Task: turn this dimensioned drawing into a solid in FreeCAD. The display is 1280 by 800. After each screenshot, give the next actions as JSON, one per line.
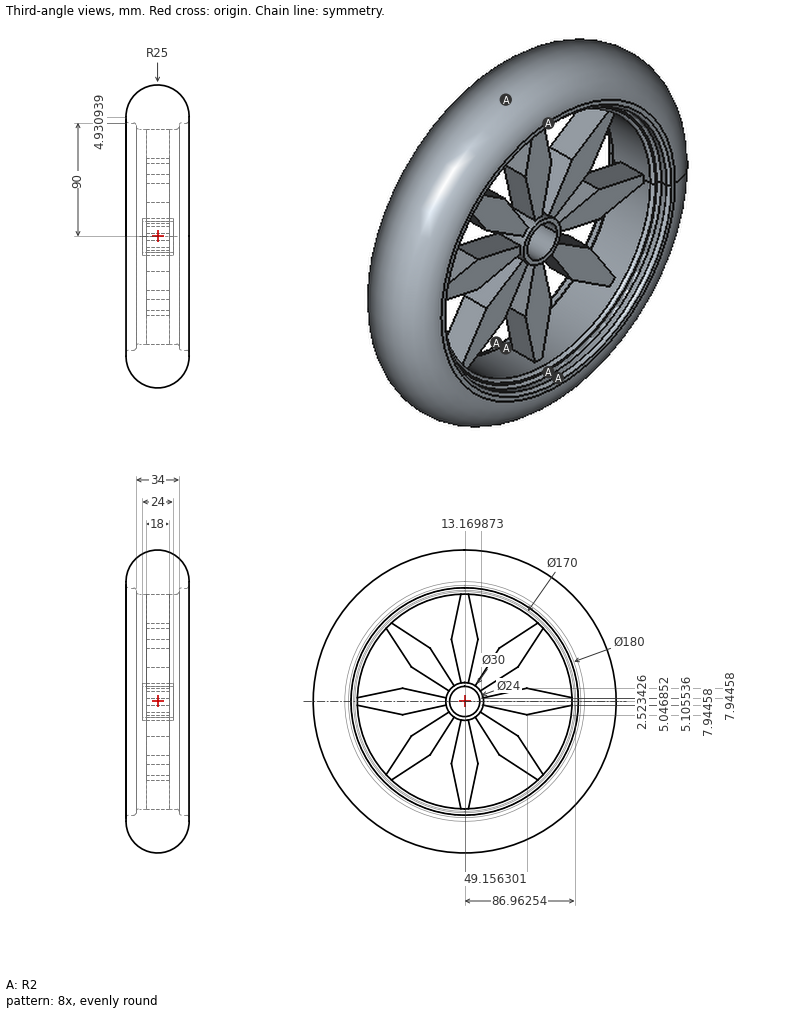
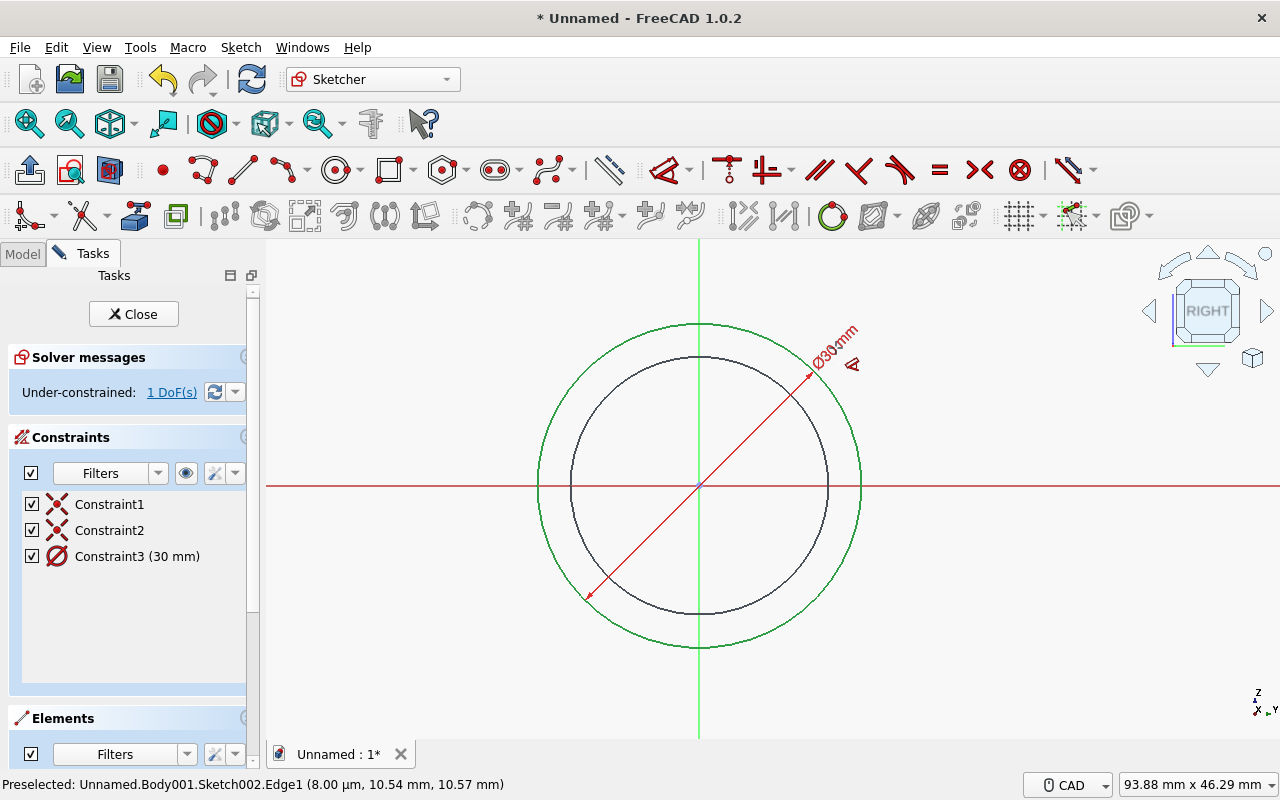
{"action": "left_click", "coordinate": [790, 394]}
{"action": "left_click", "coordinate": [876, 433]}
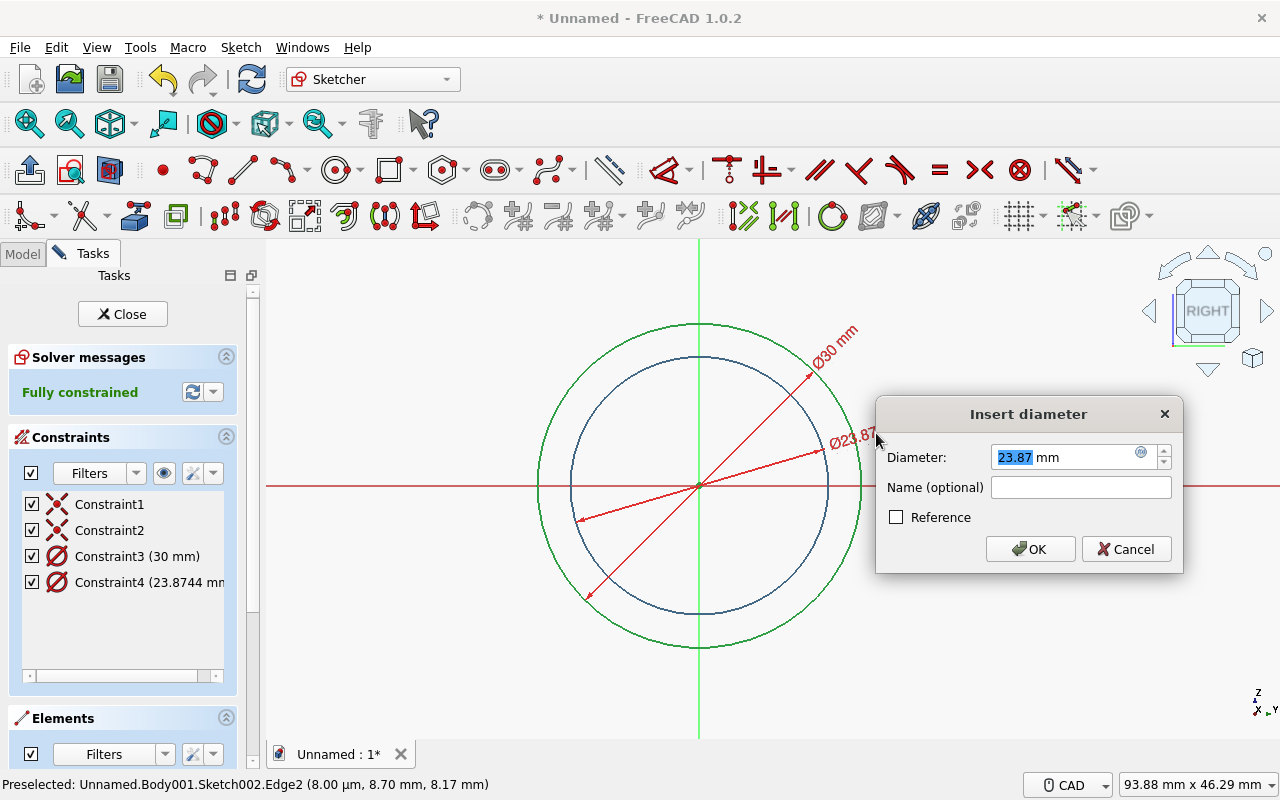
{"action": "type", "text": "24"}
{"action": "key", "text": "Return"}
{"action": "key", "text": "Escape"}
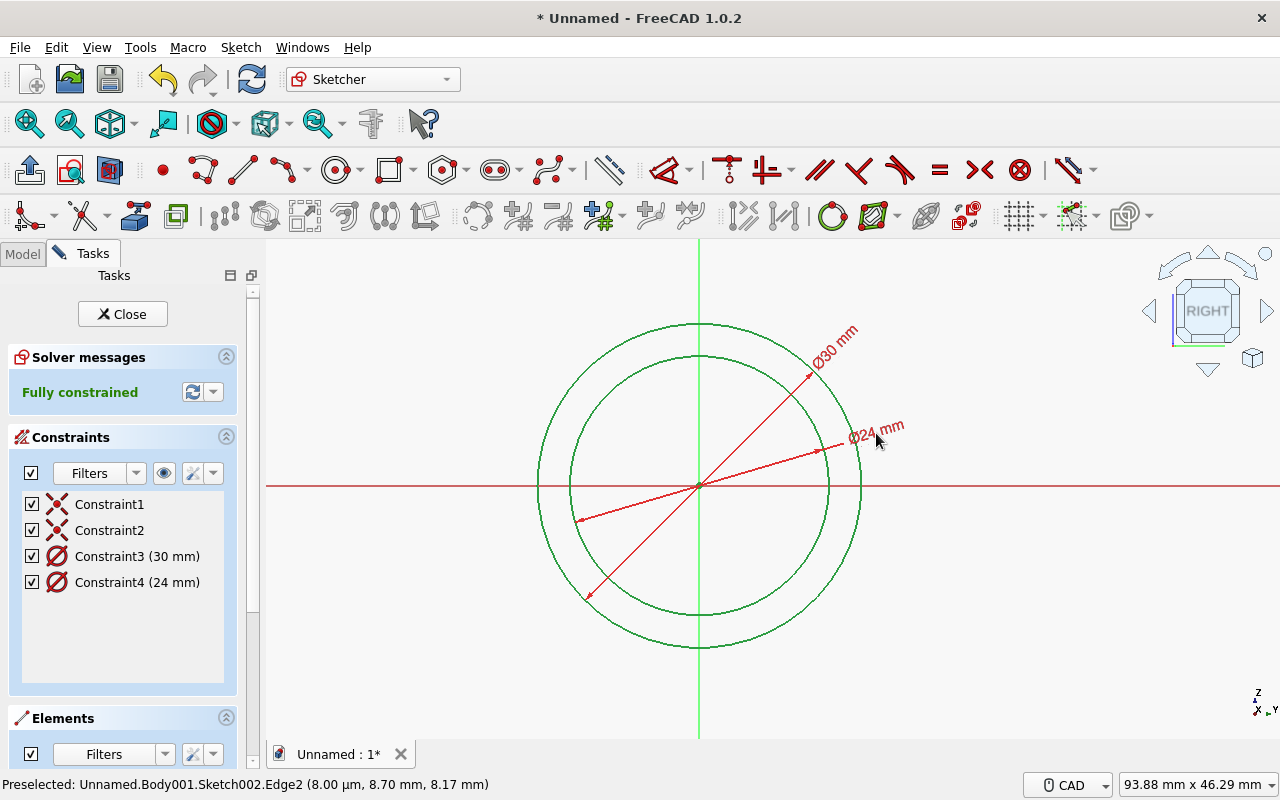
{"action": "left_click", "coordinate": [123, 314]}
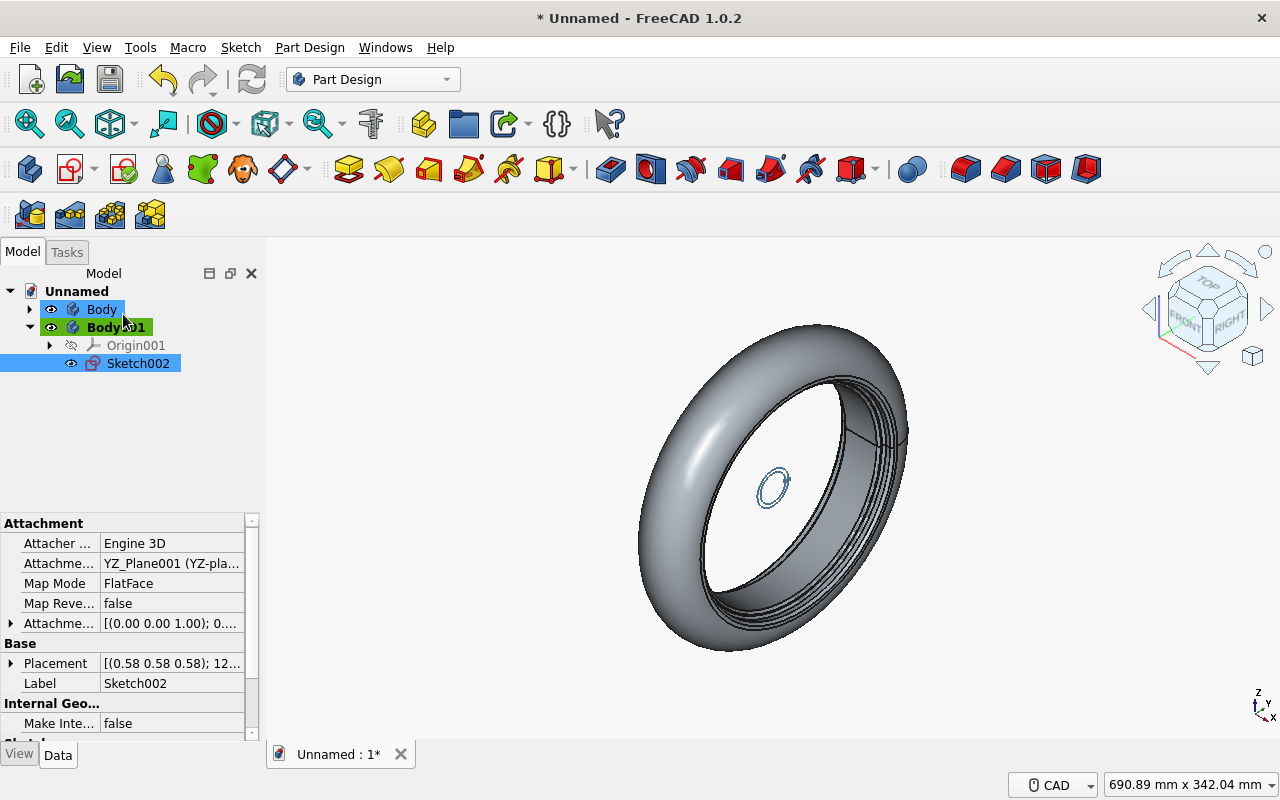
{"action": "left_click", "coordinate": [350, 170]}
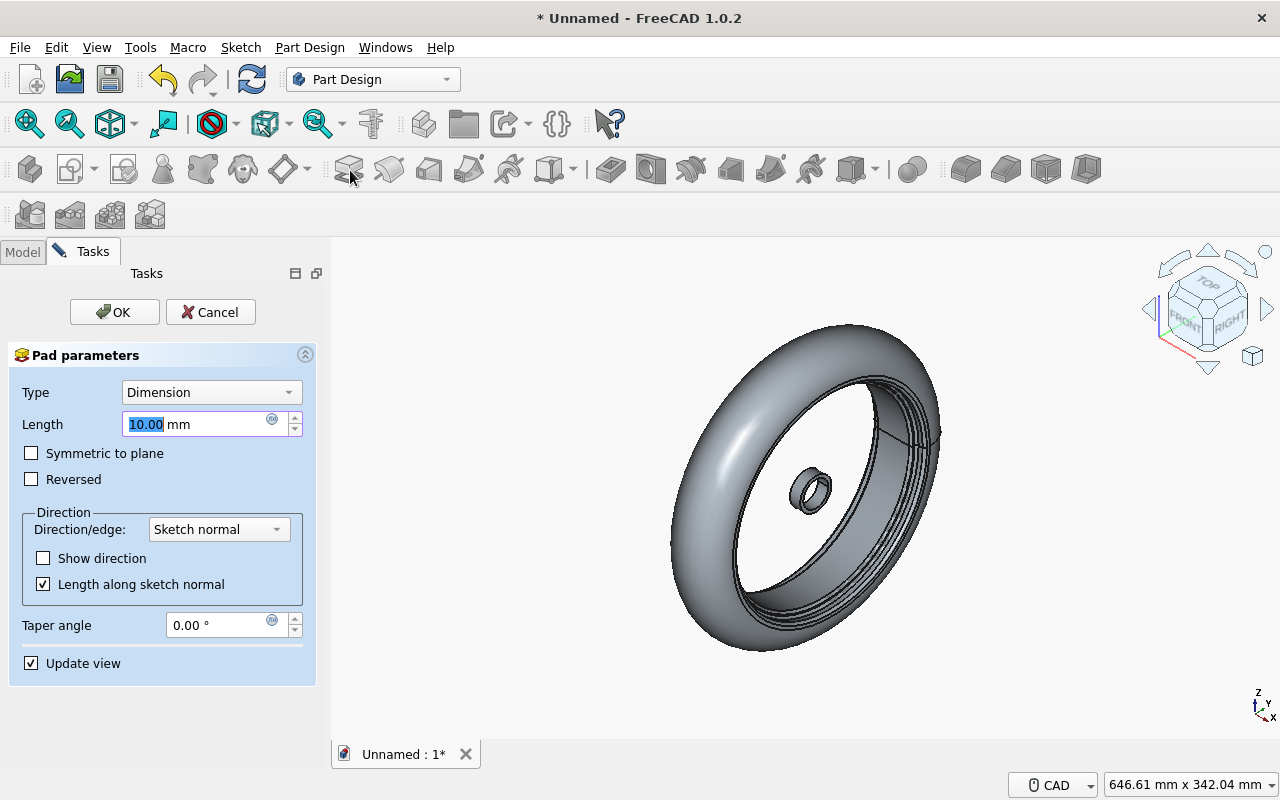
{"action": "type", "text": "24"}
{"action": "key", "text": "Tab"}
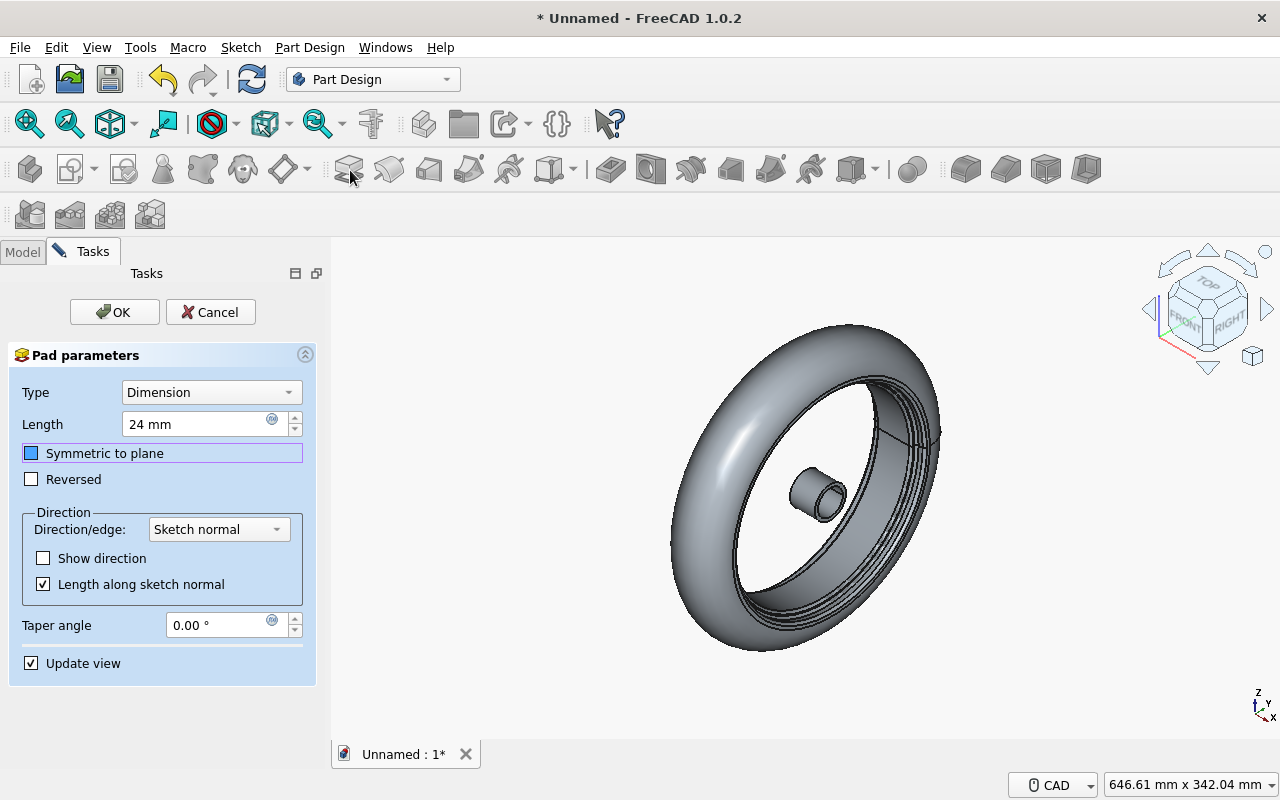
{"action": "left_click", "coordinate": [30, 453]}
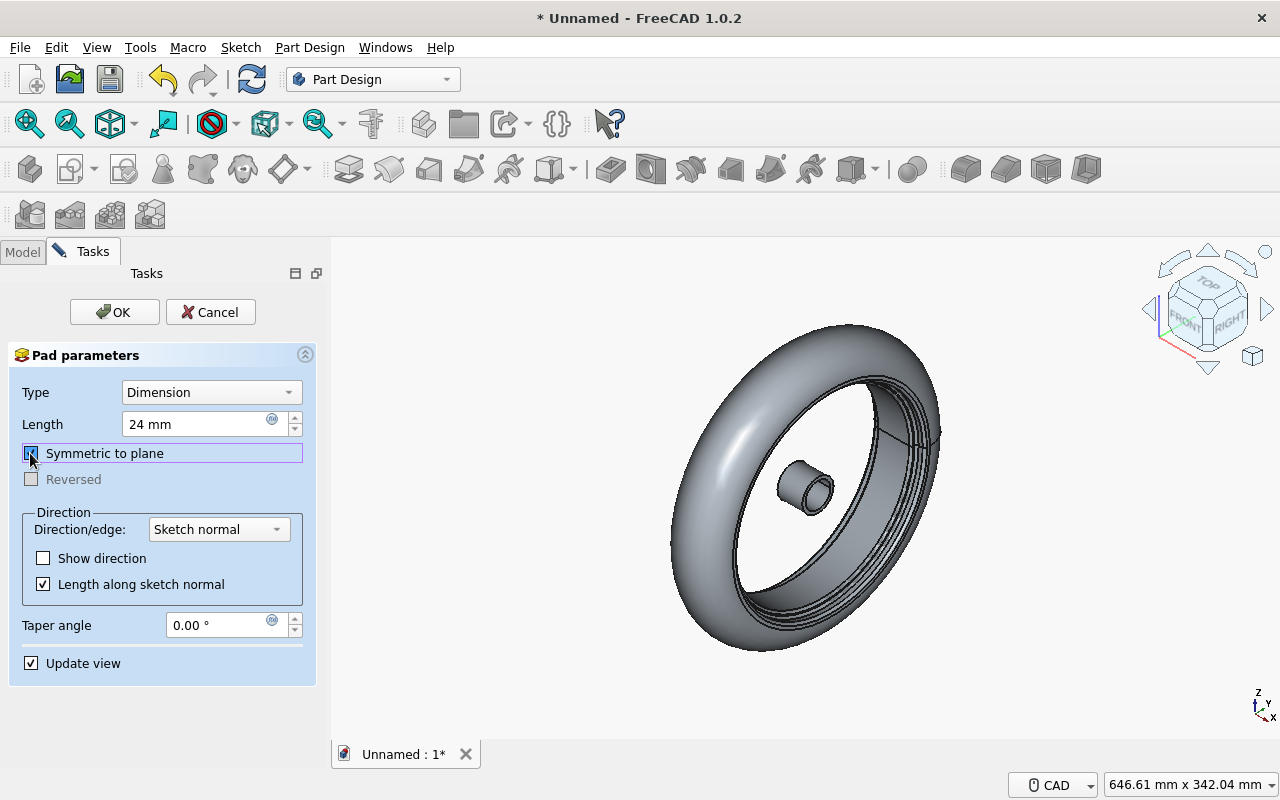
{"action": "left_click", "coordinate": [115, 312]}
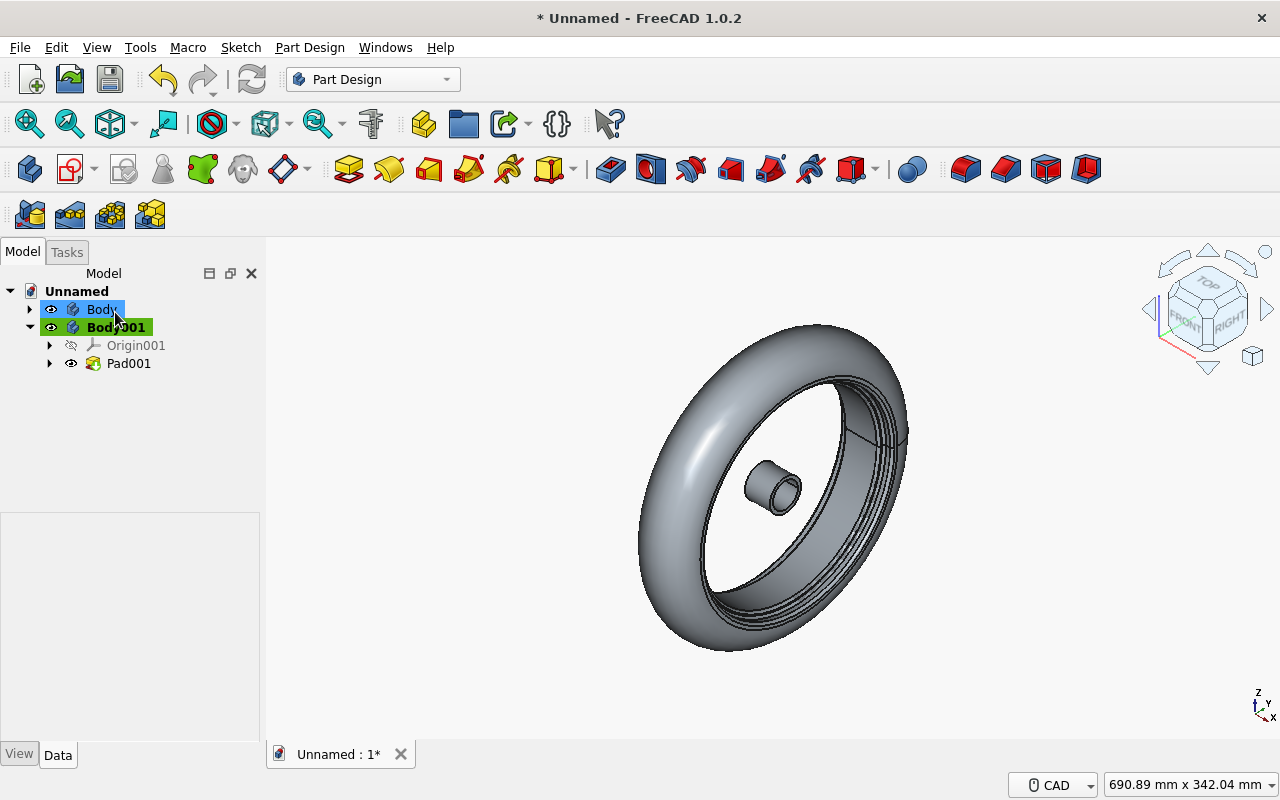
{"action": "key", "text": "v f"}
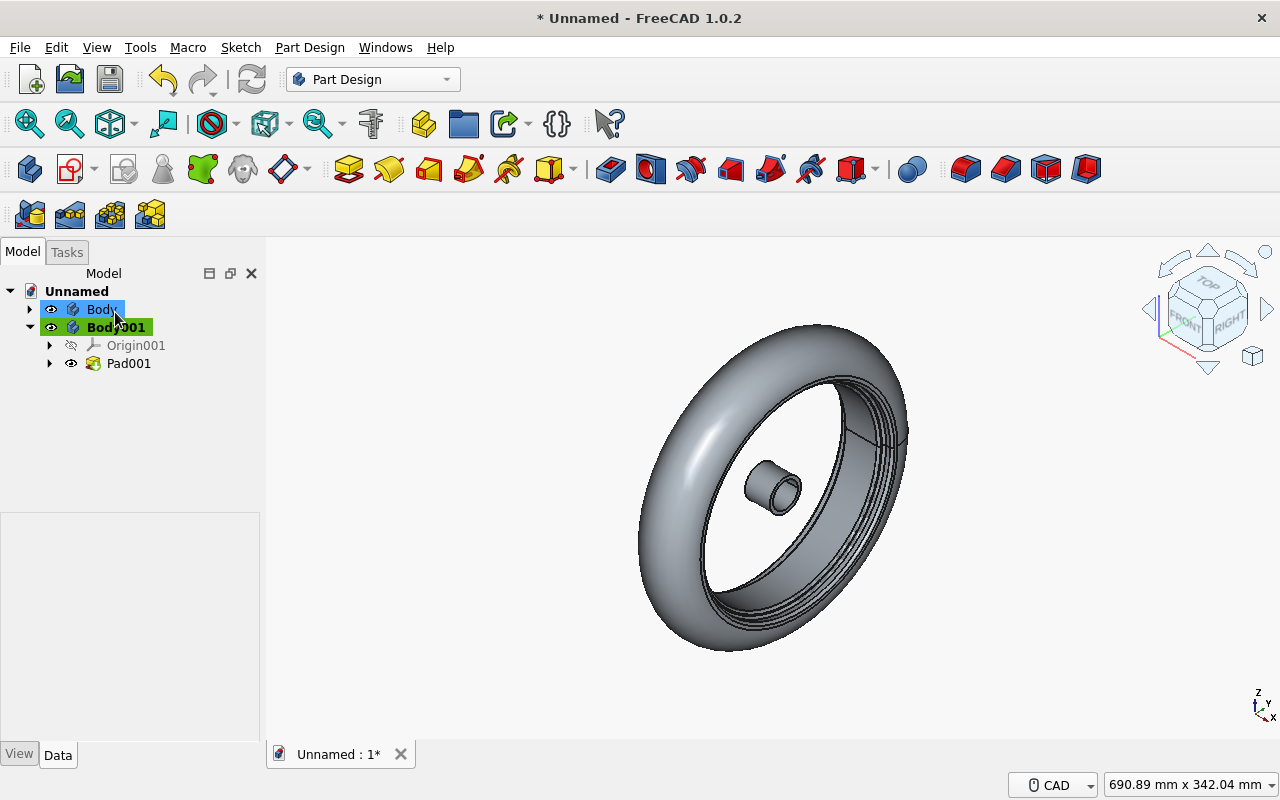
{"action": "double_click", "coordinate": [96, 309]}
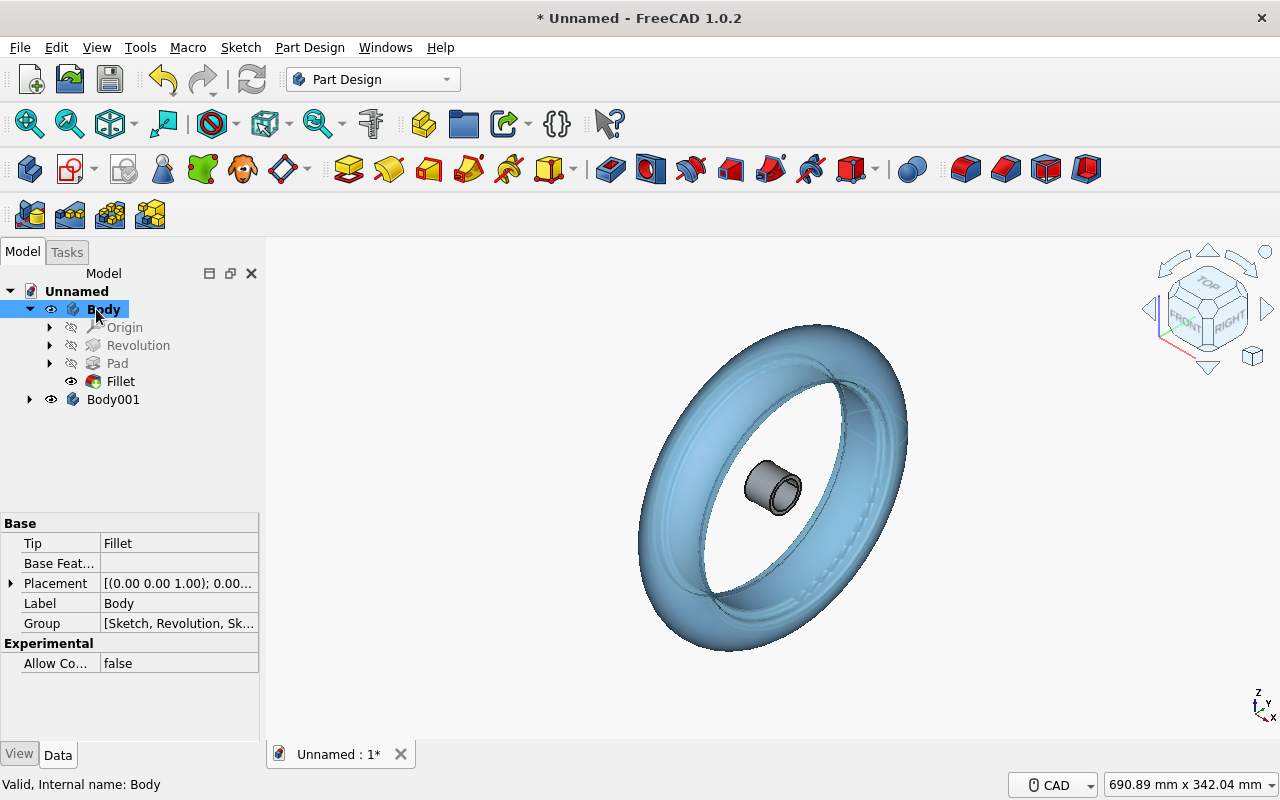
{"action": "left_click", "coordinate": [96, 309]}